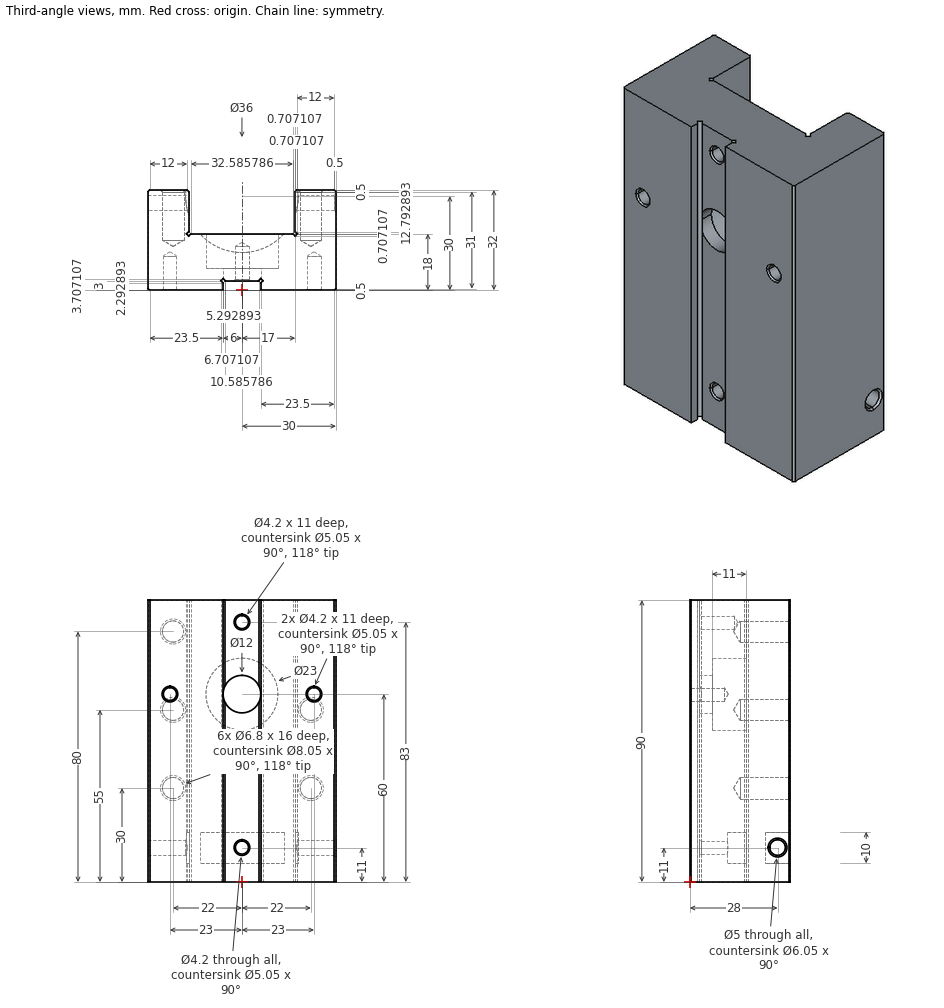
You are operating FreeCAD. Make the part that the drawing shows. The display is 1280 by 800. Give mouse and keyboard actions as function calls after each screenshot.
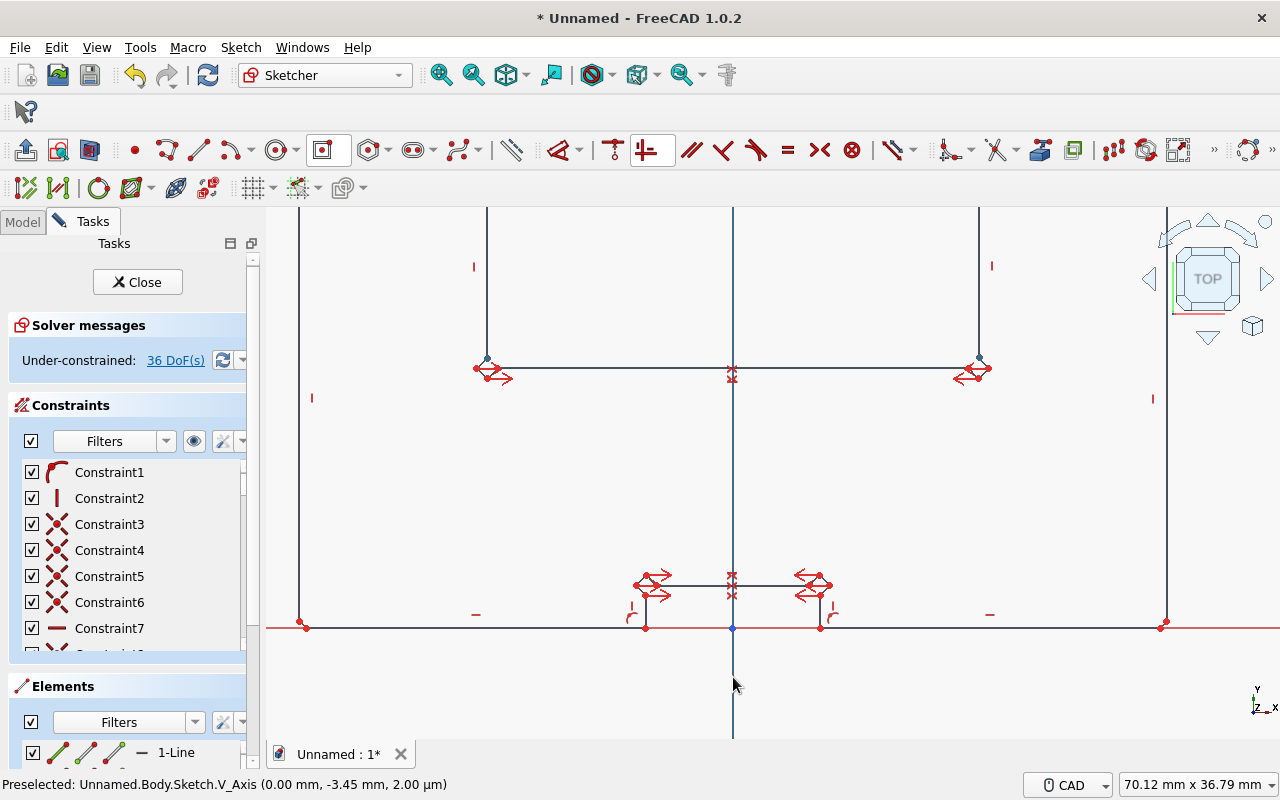
click(820, 150)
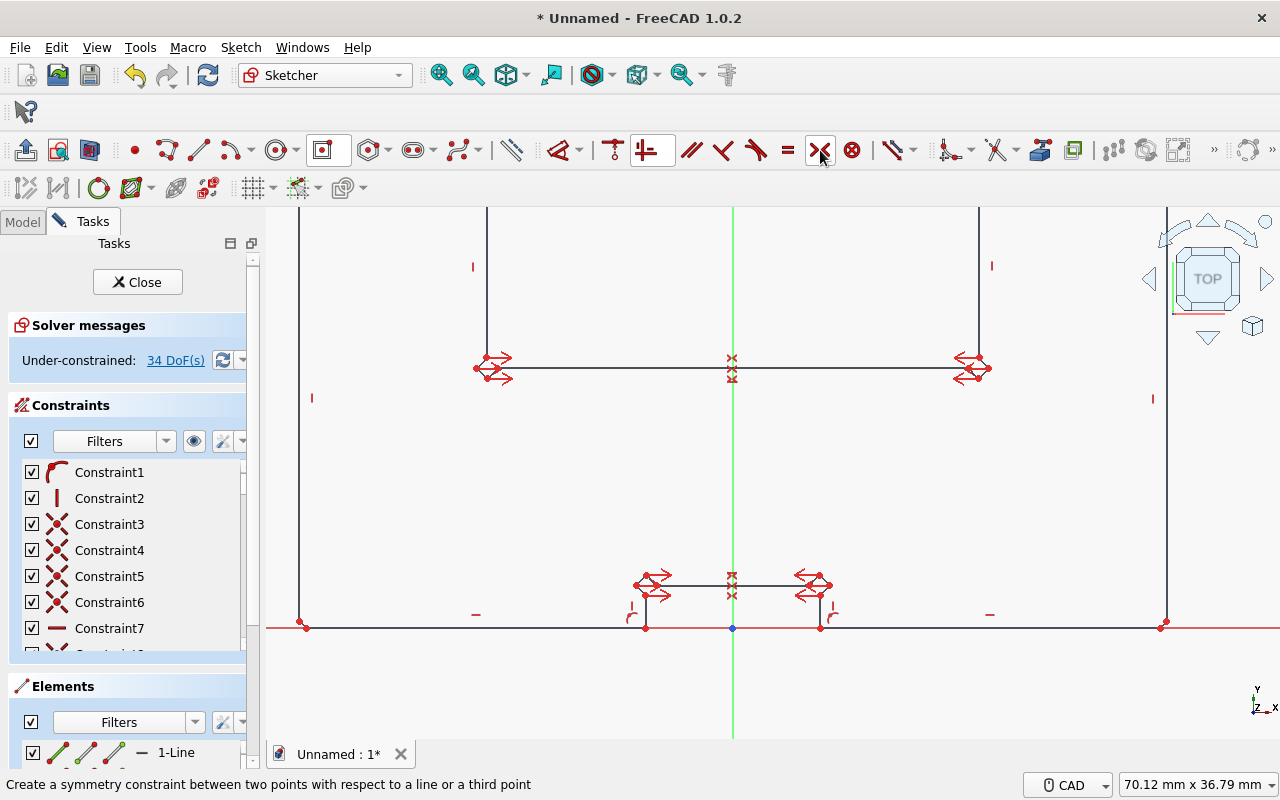
scroll(647, 628, down, 2)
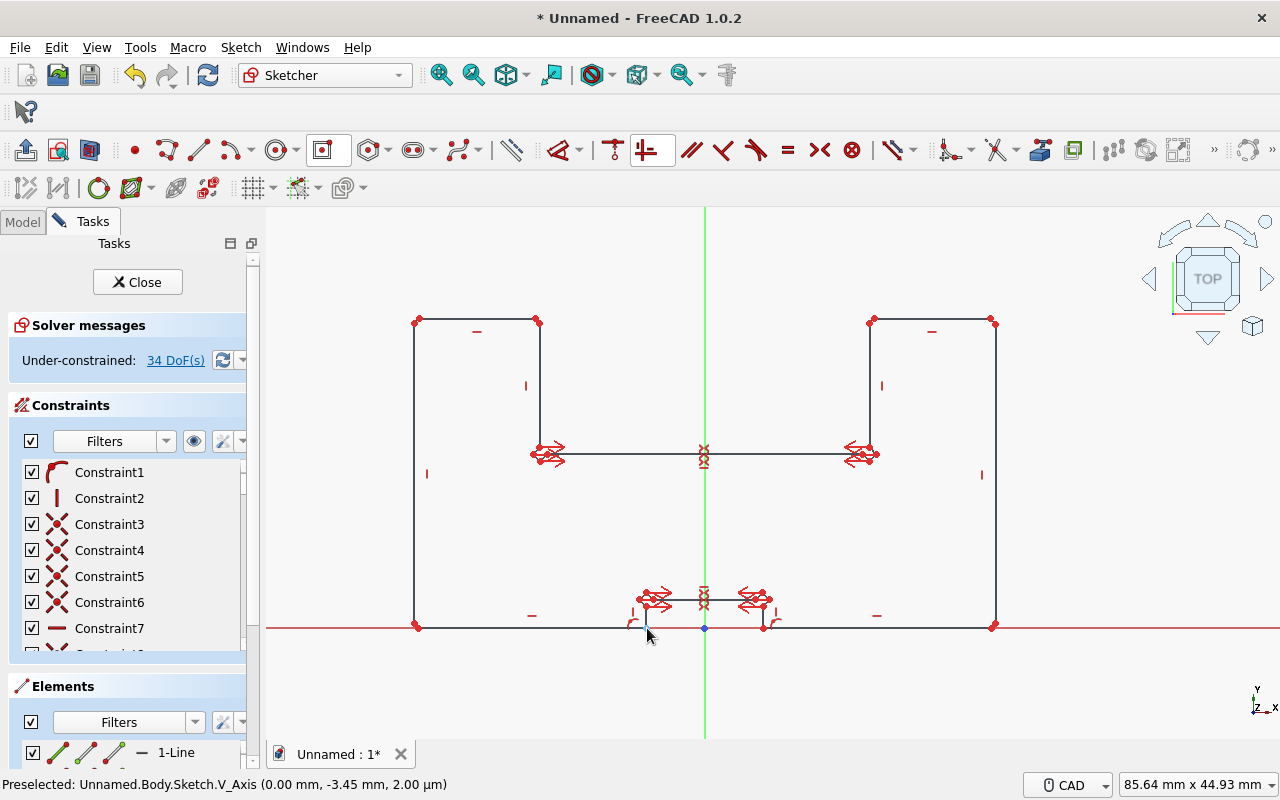
scroll(874, 318, up, 3)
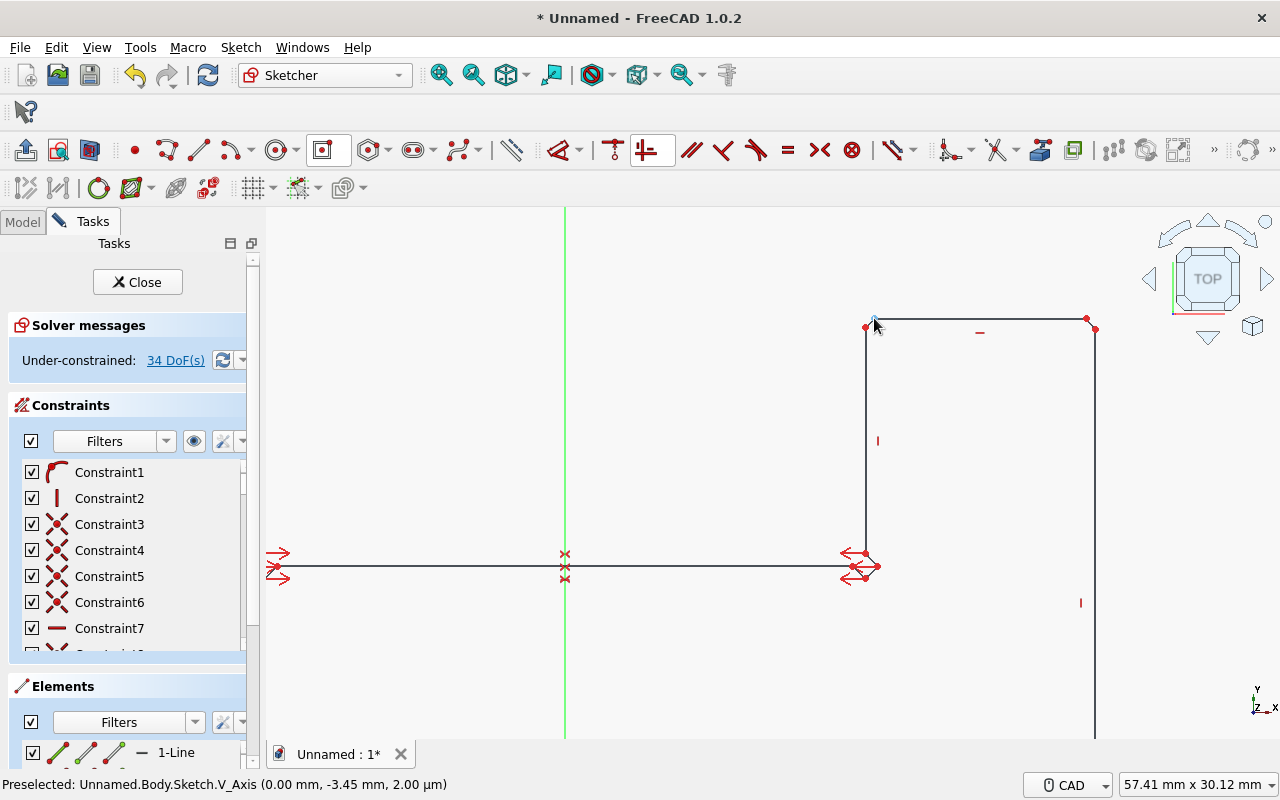
click(874, 319)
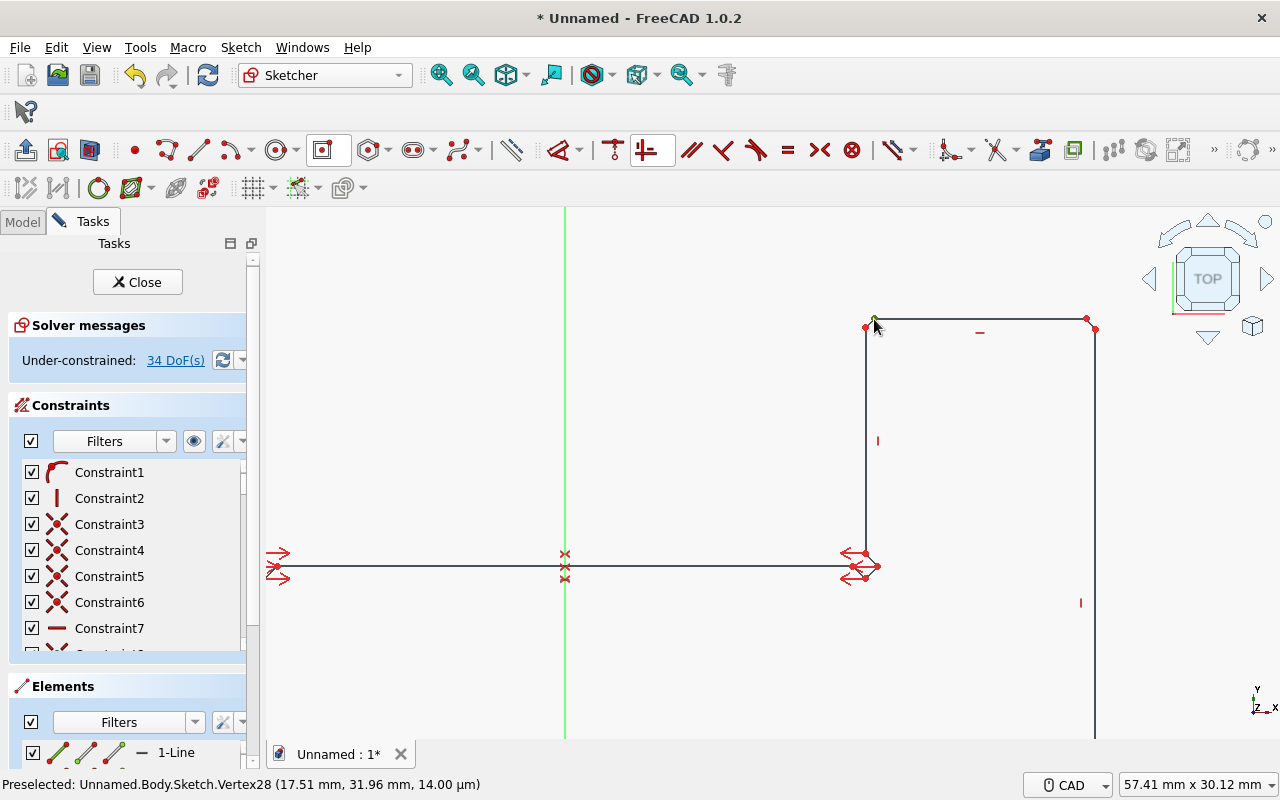
scroll(874, 318, down, 3)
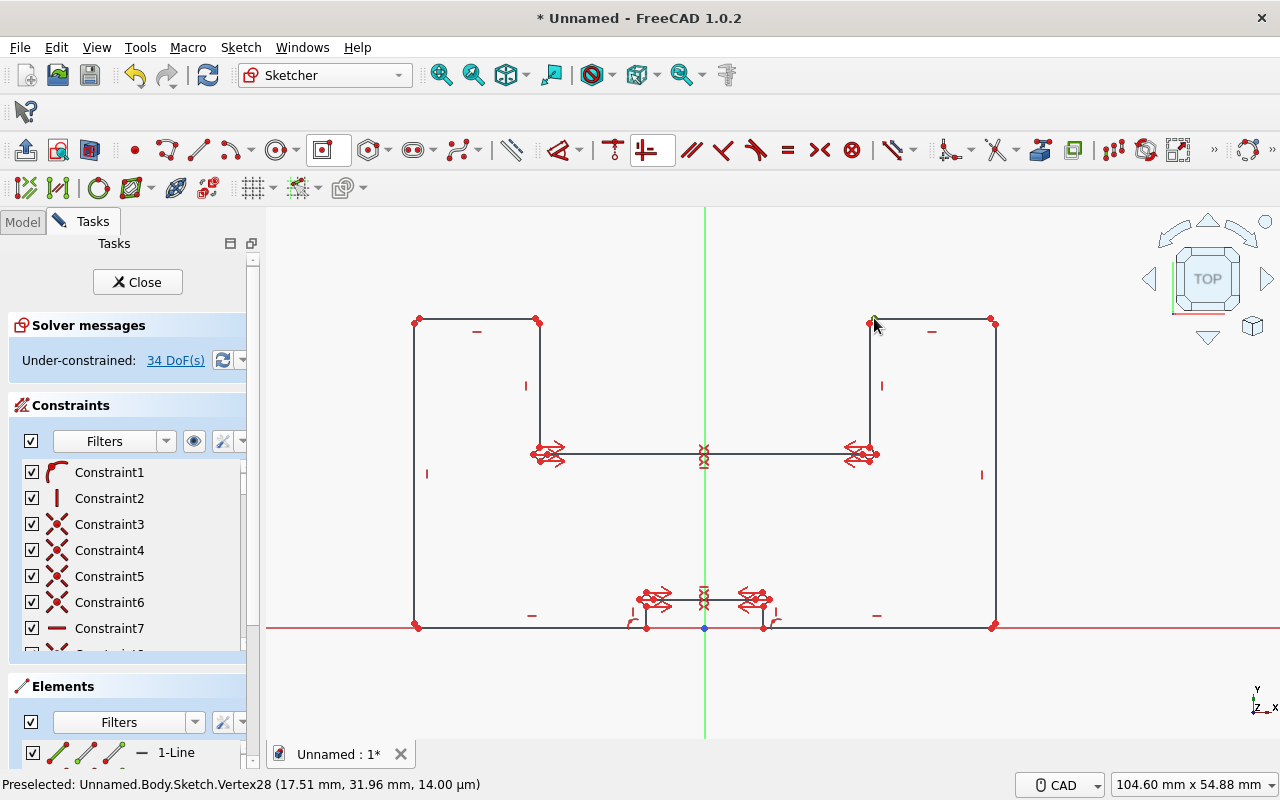
scroll(535, 318, up, 3)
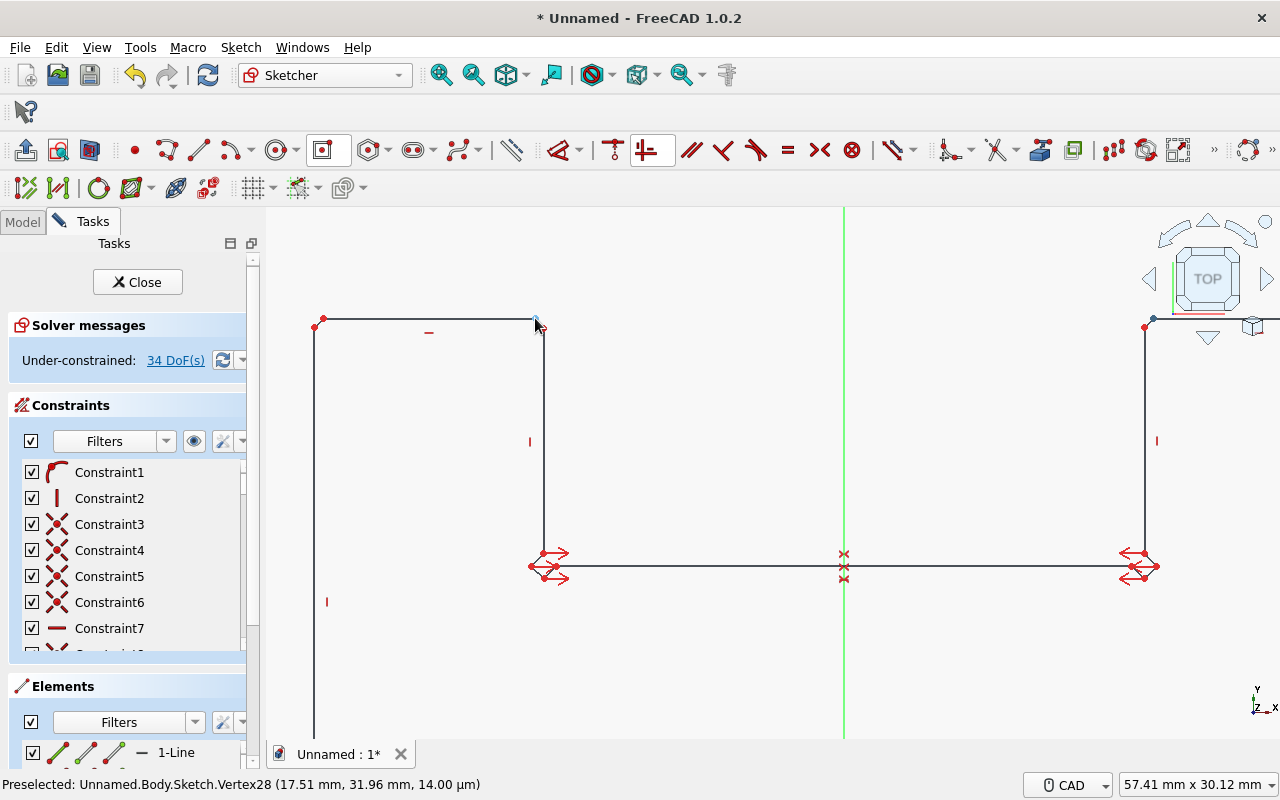
click(535, 319)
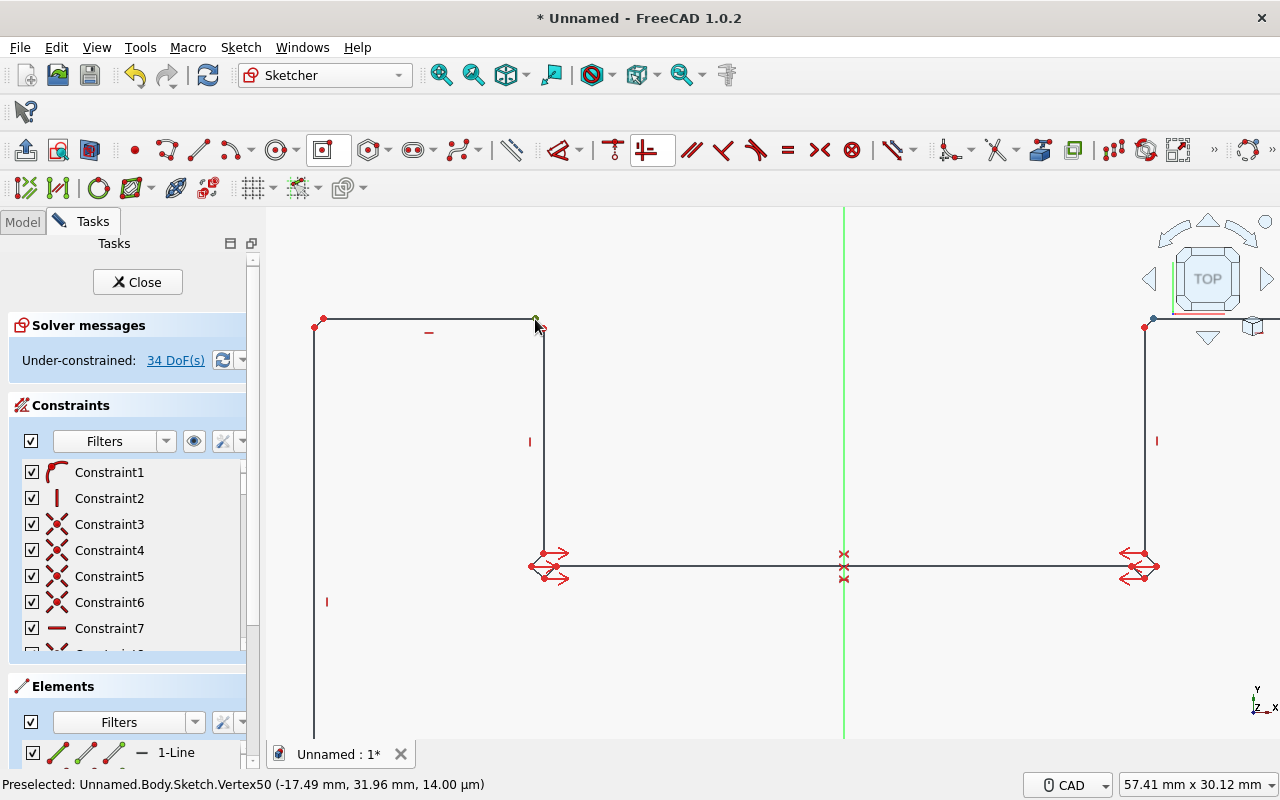
click(844, 677)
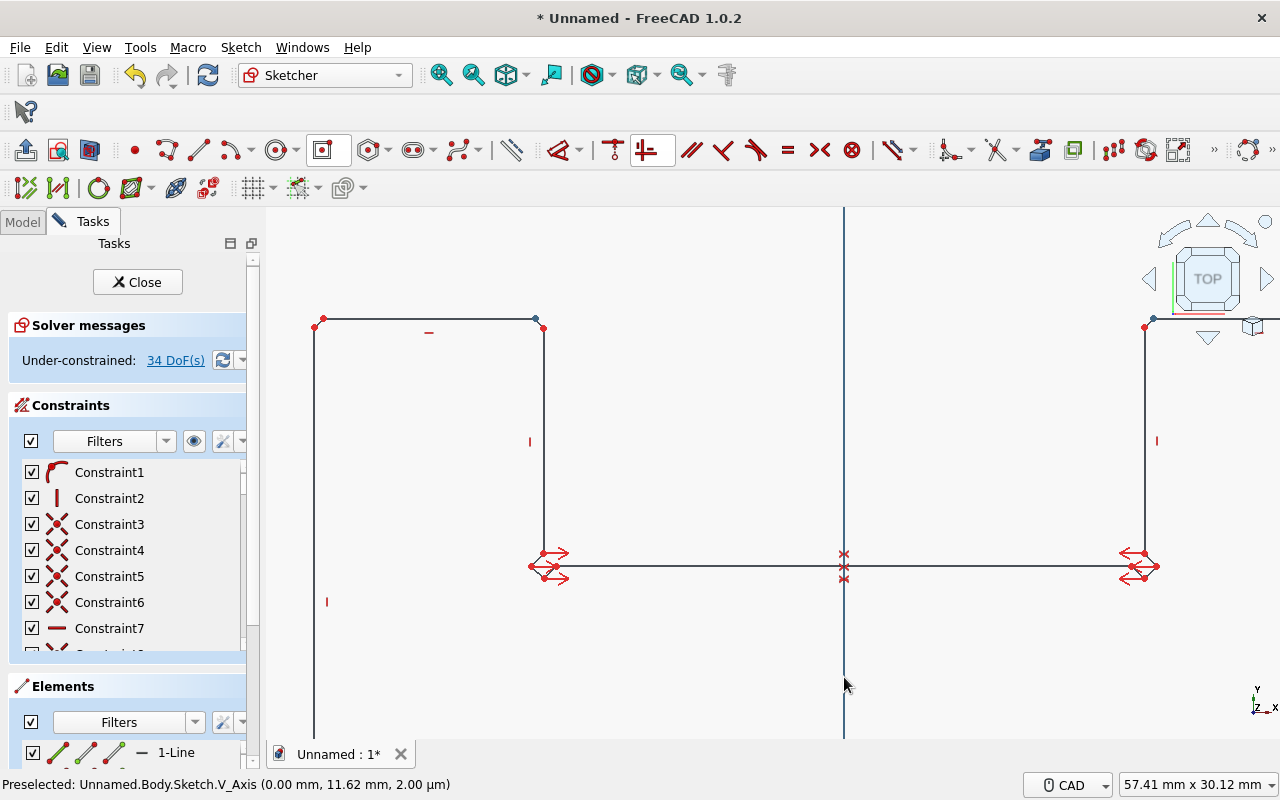
click(820, 150)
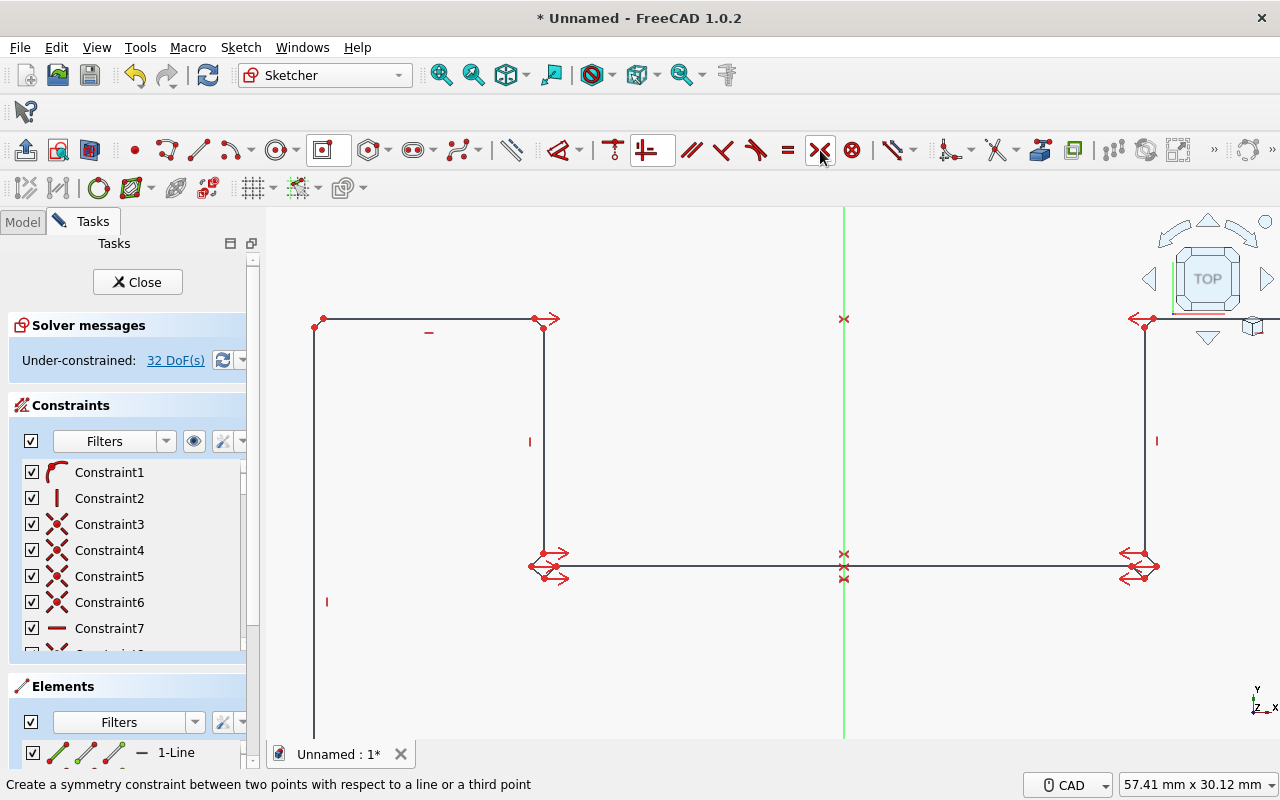
scroll(535, 318, down, 3)